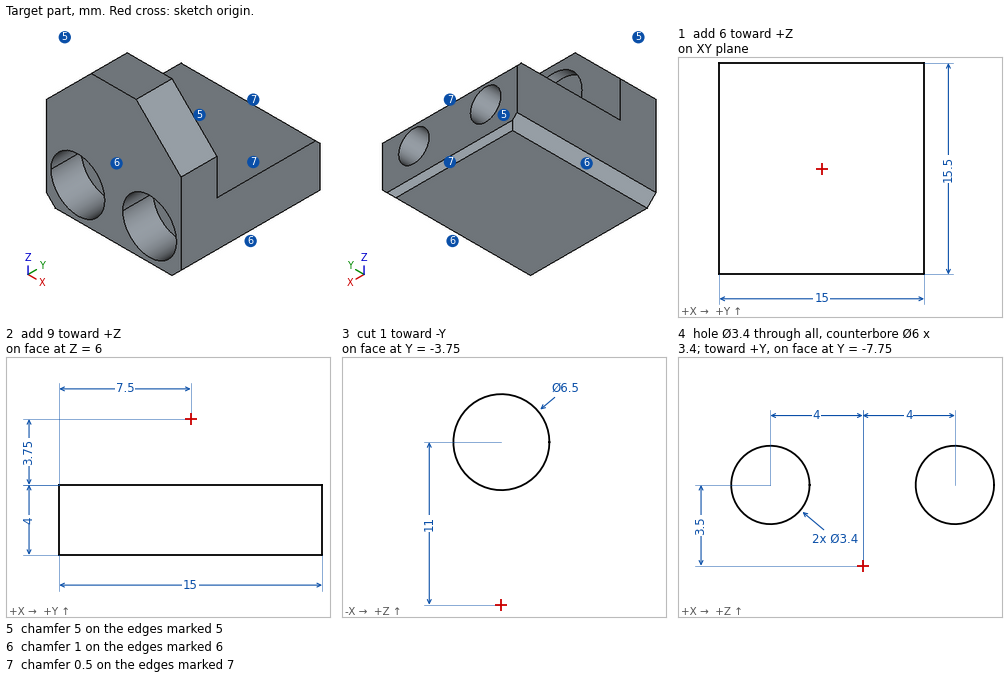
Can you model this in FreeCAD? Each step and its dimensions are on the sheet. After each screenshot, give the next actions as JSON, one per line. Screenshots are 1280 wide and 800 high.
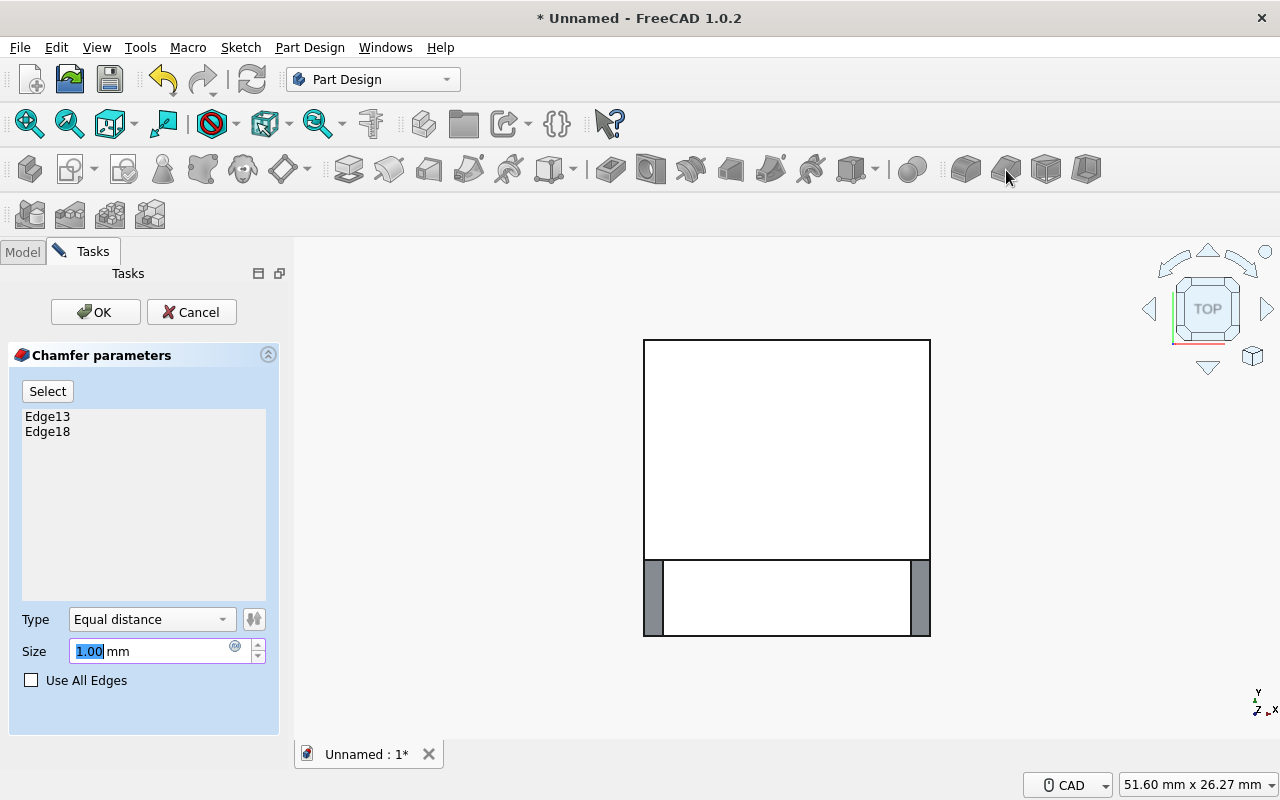
{"action": "type", "text": "5"}
{"action": "key", "text": "Tab"}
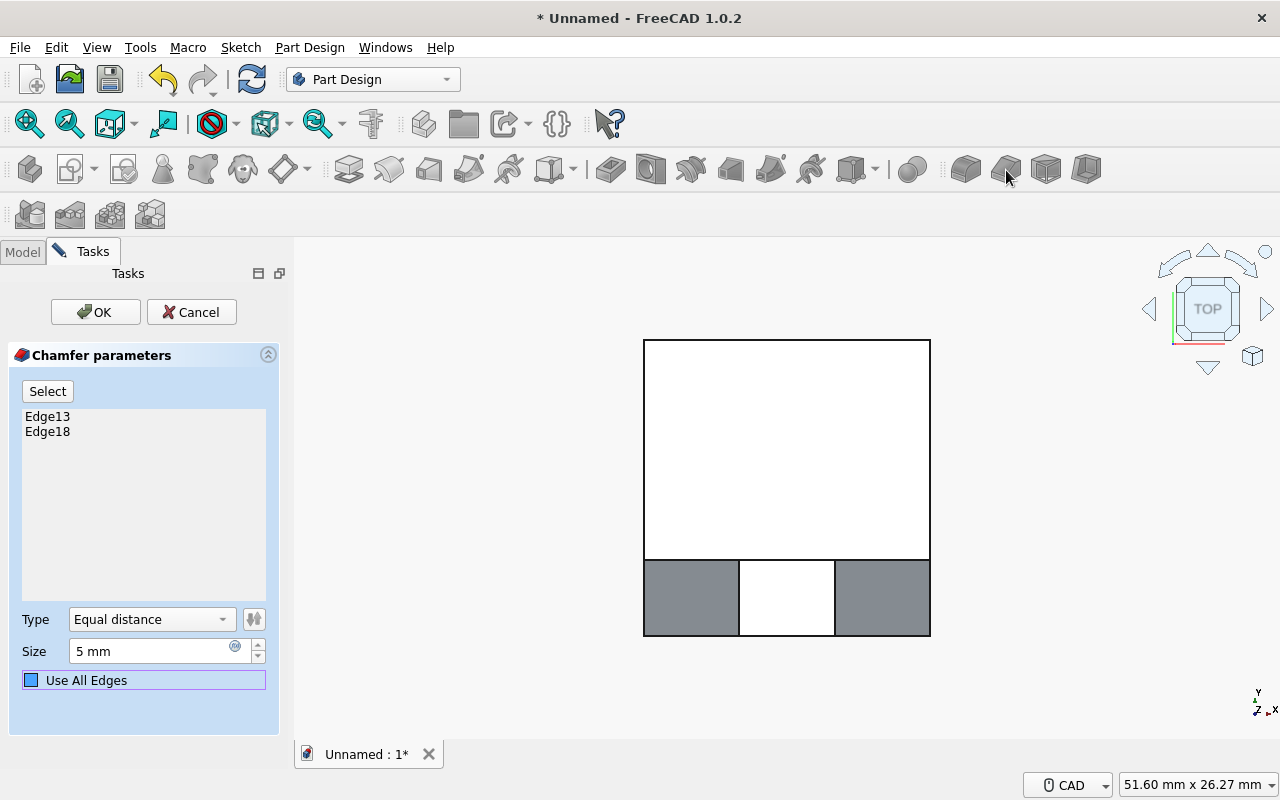
{"action": "left_click", "coordinate": [96, 312]}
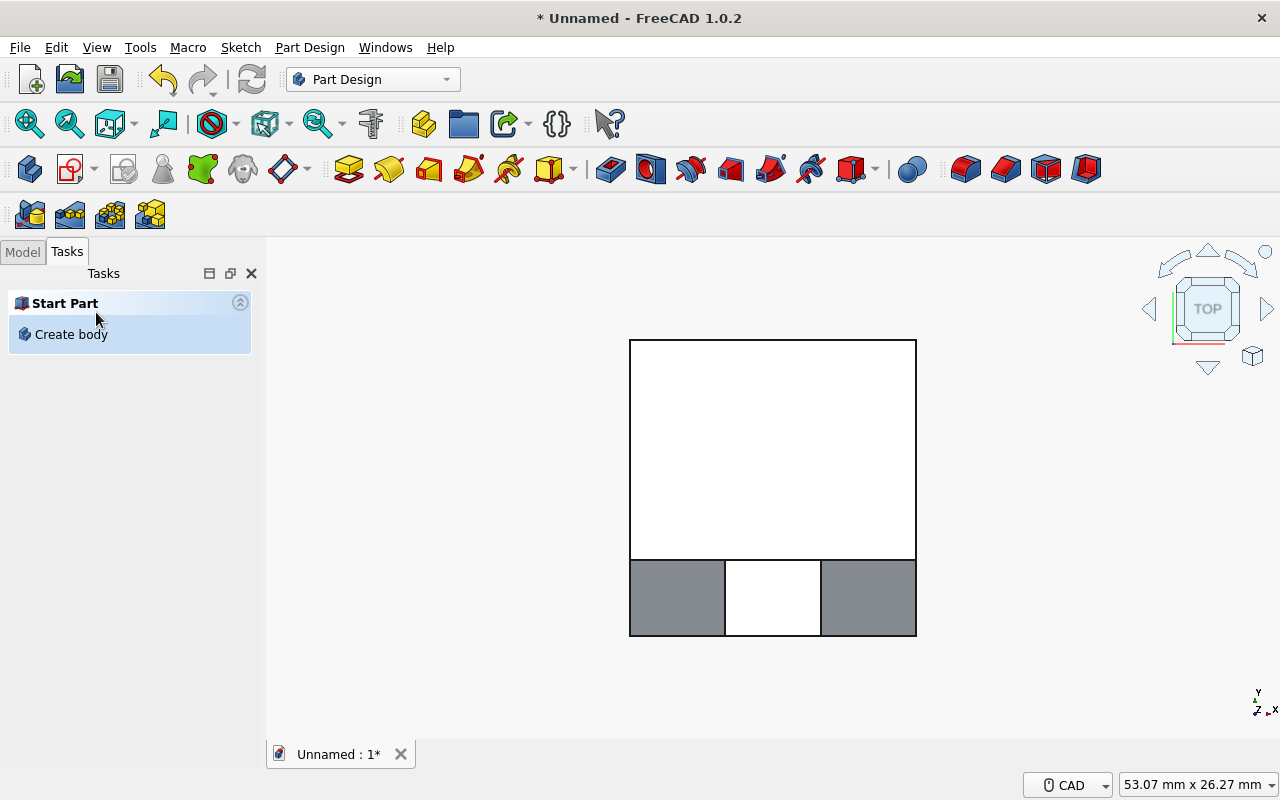
{"action": "key", "text": "0"}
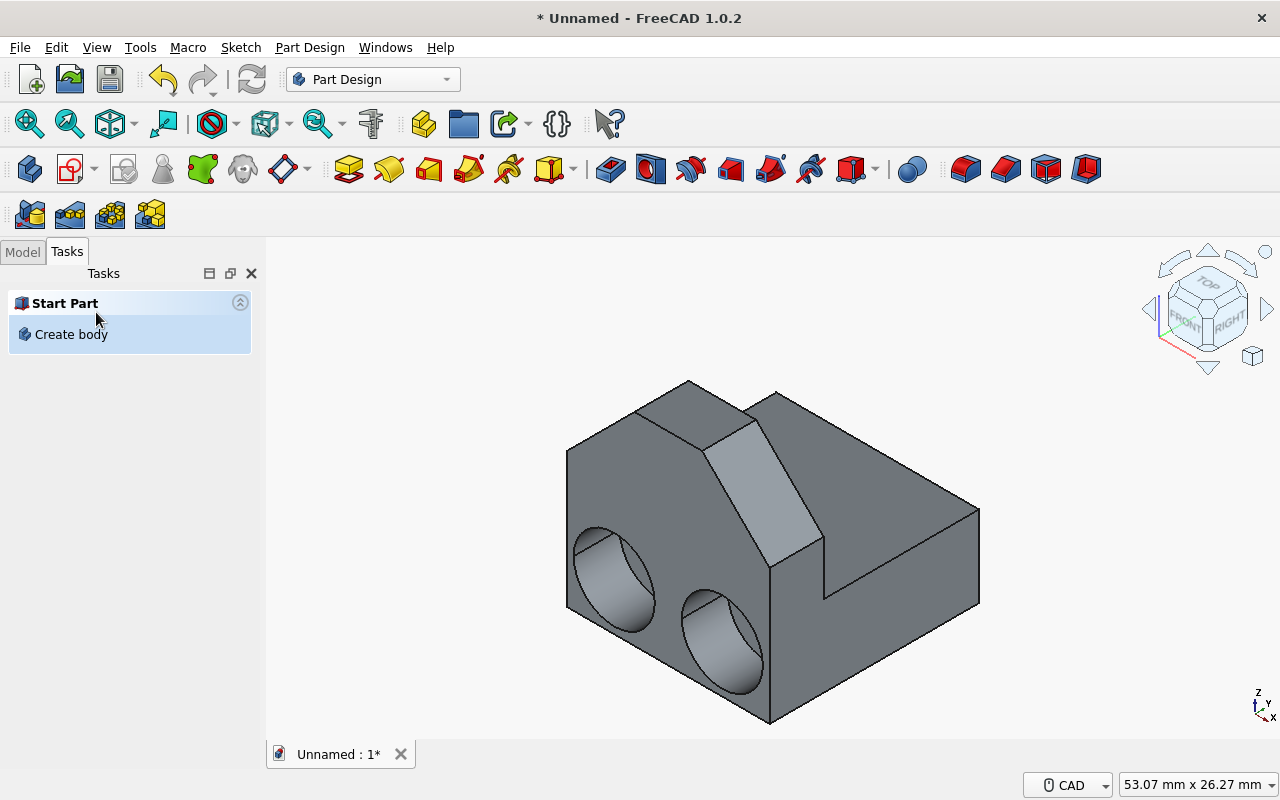
{"action": "key", "text": "2"}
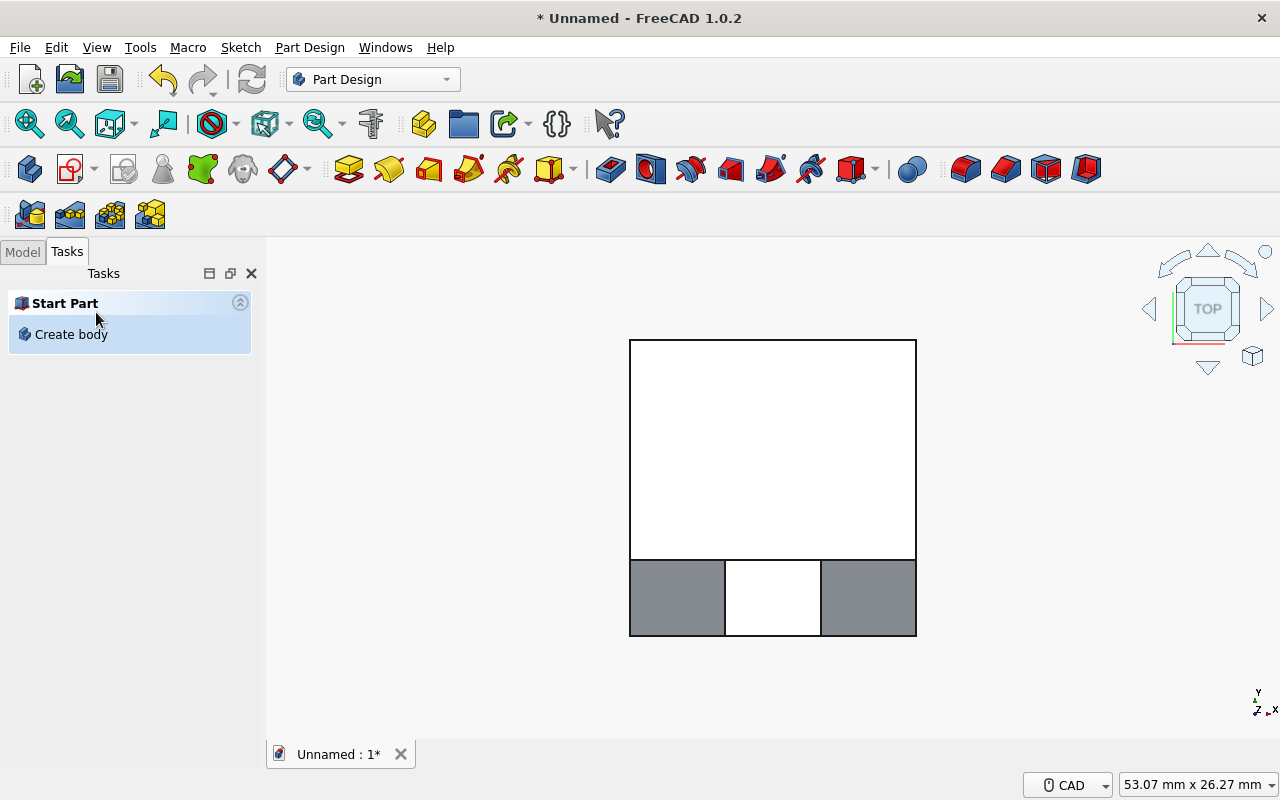
{"action": "key", "text": "1"}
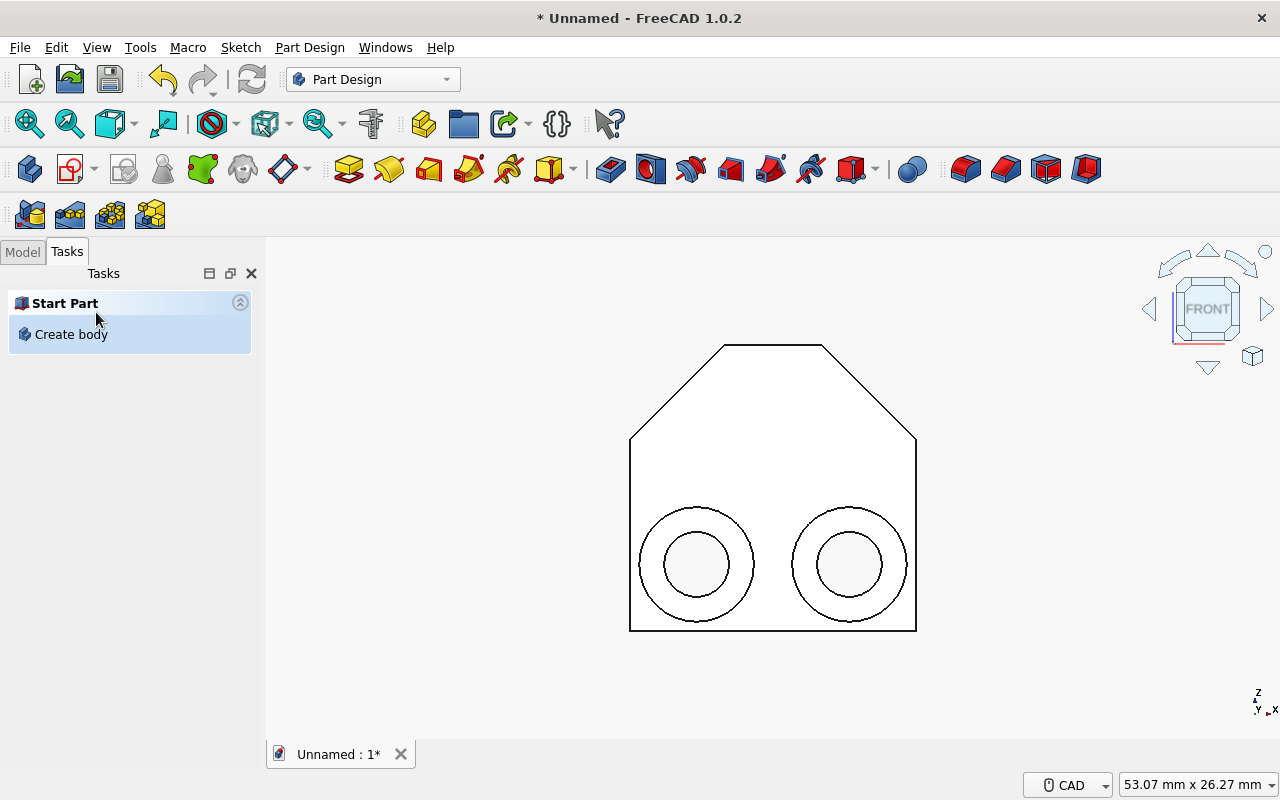
{"action": "key", "text": "3"}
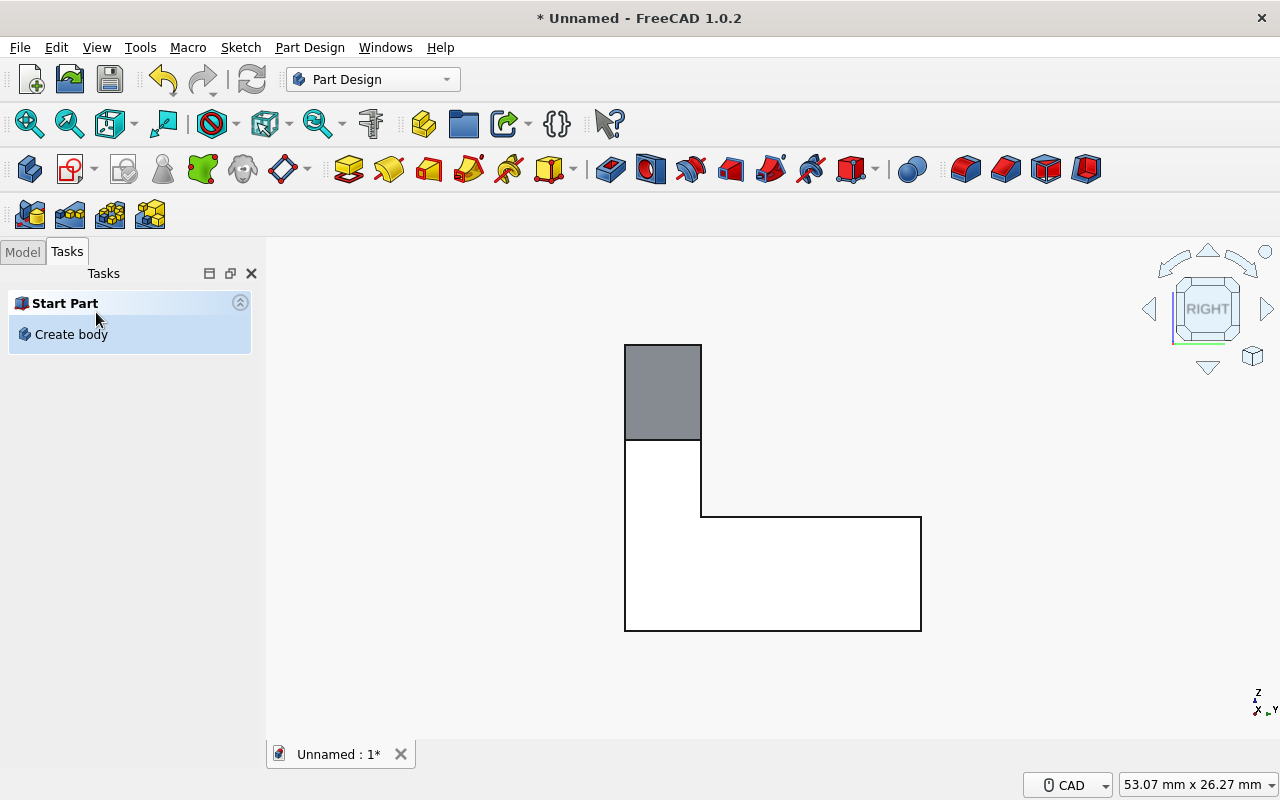
{"action": "left_click", "coordinate": [773, 630]}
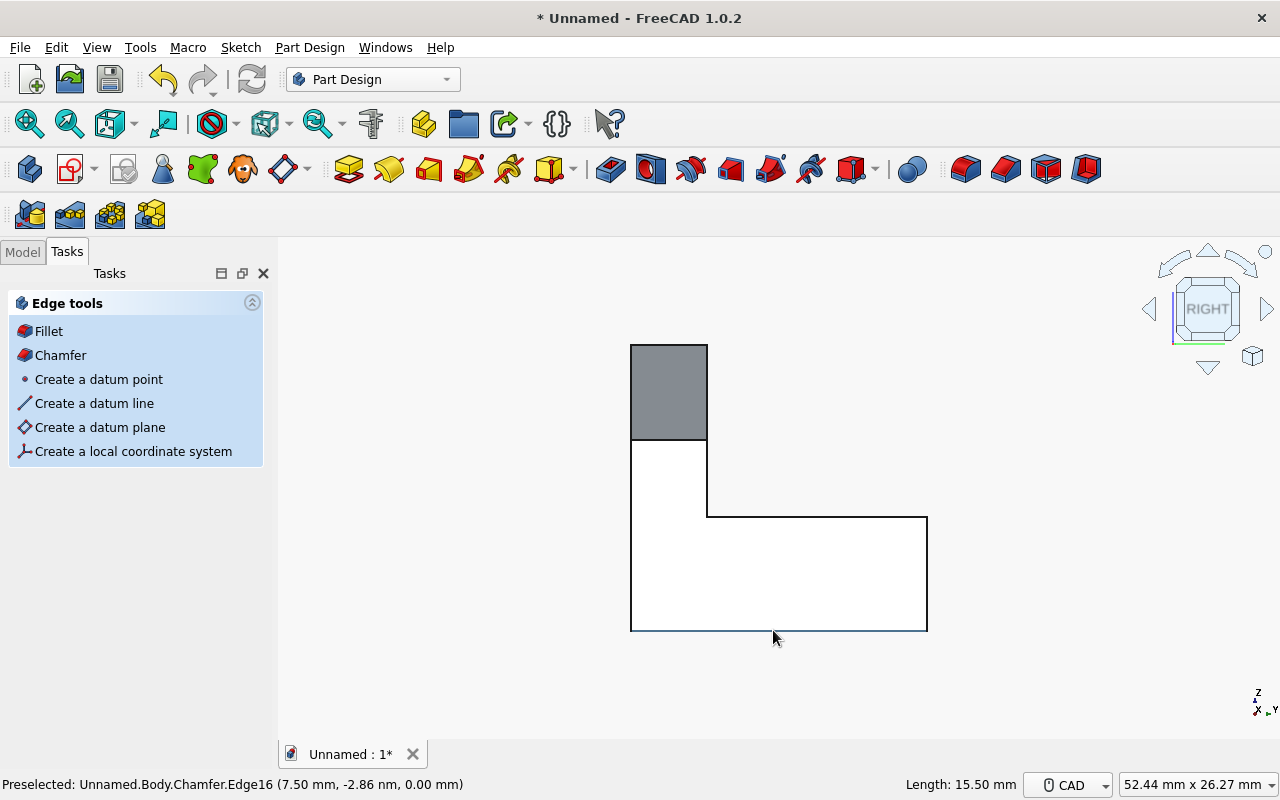
{"action": "key", "text": "5"}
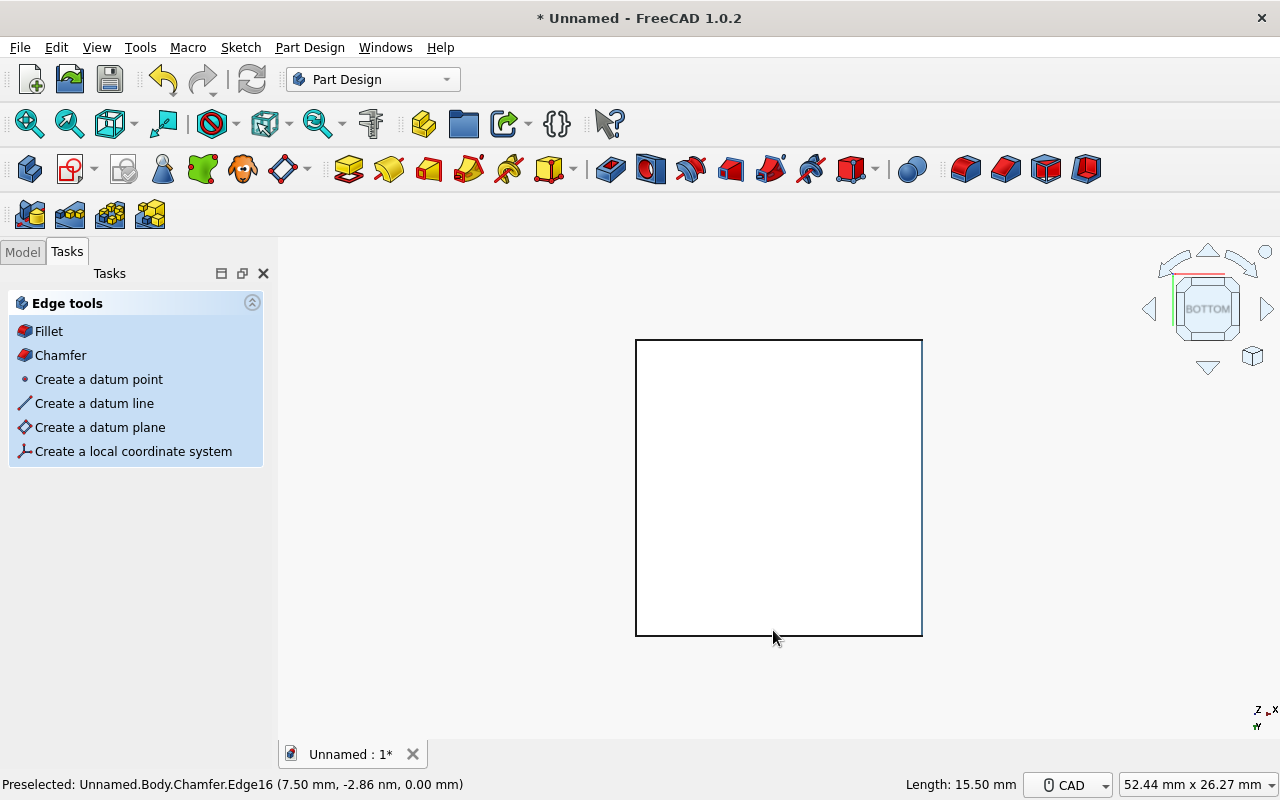
{"action": "left_click", "coordinate": [636, 487], "text": "ctrl"}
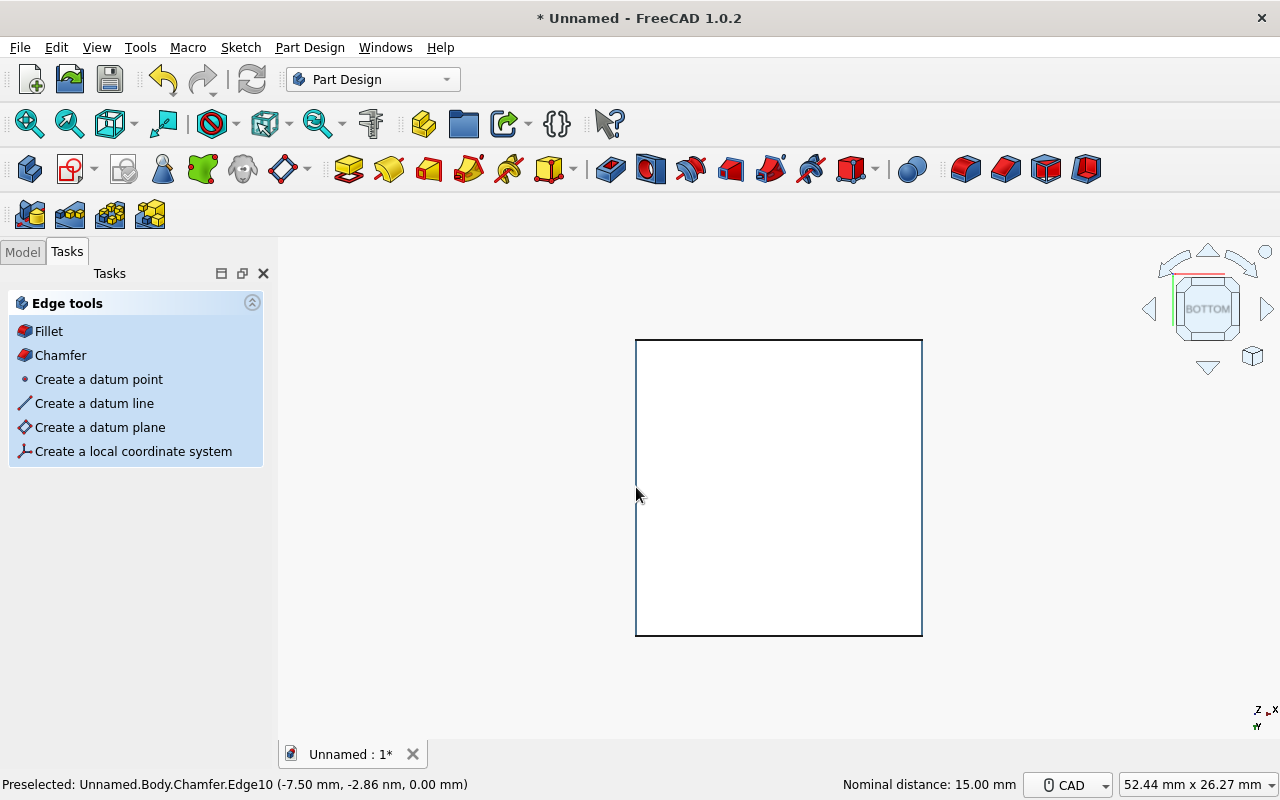
{"action": "left_click", "coordinate": [1006, 170]}